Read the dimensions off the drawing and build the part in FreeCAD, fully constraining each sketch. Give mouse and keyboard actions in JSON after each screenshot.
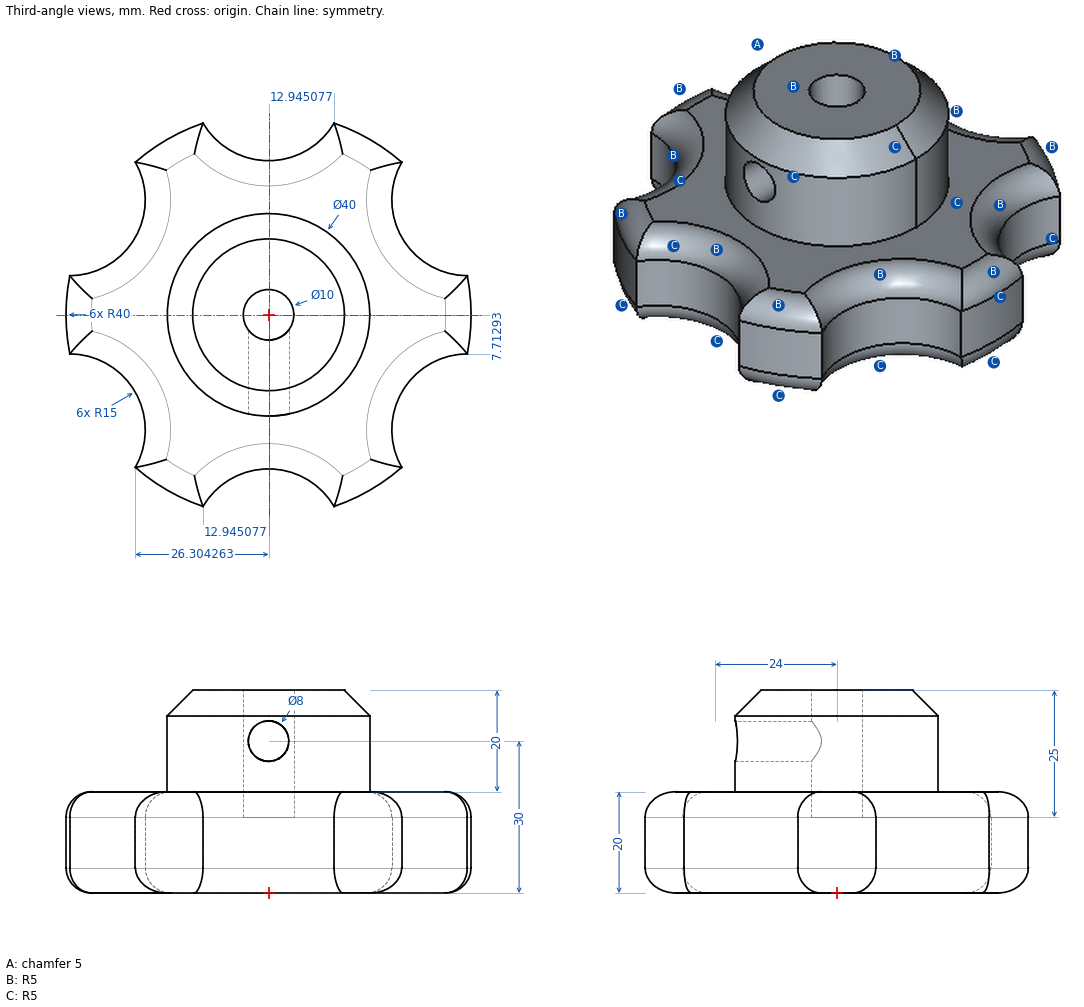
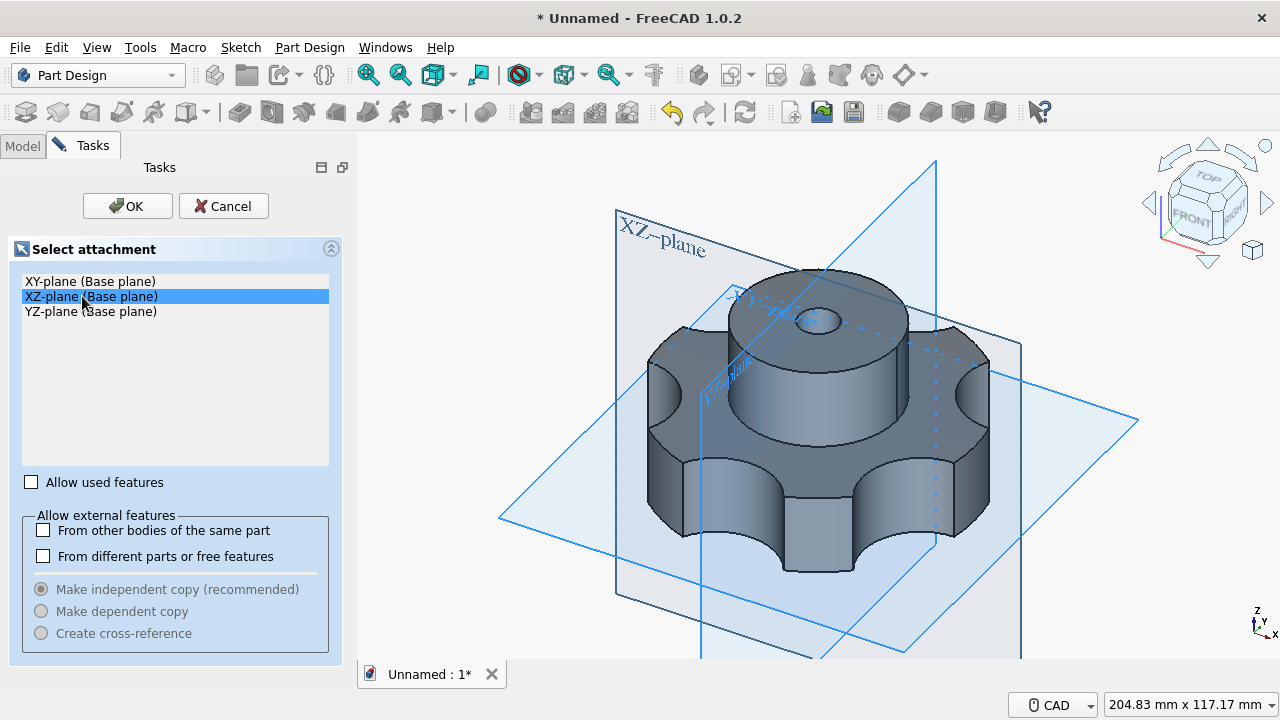
{"action": "left_click", "coordinate": [128, 206]}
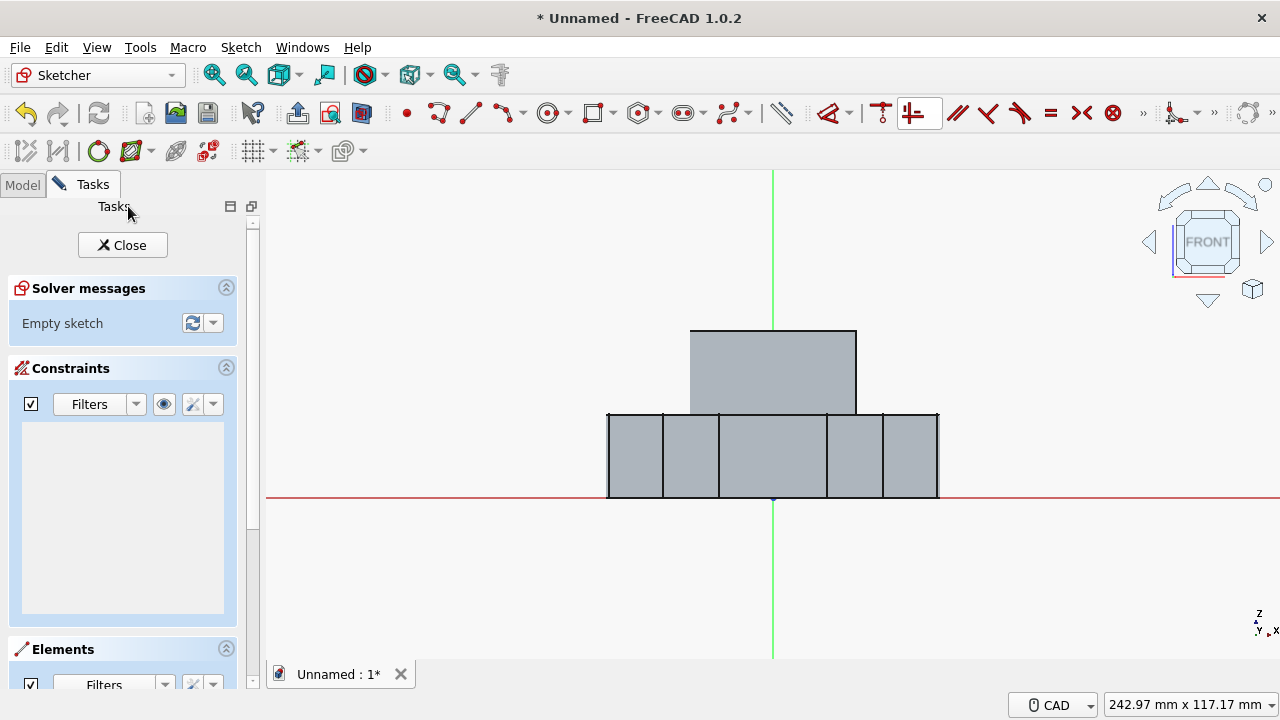
{"action": "left_click", "coordinate": [362, 114]}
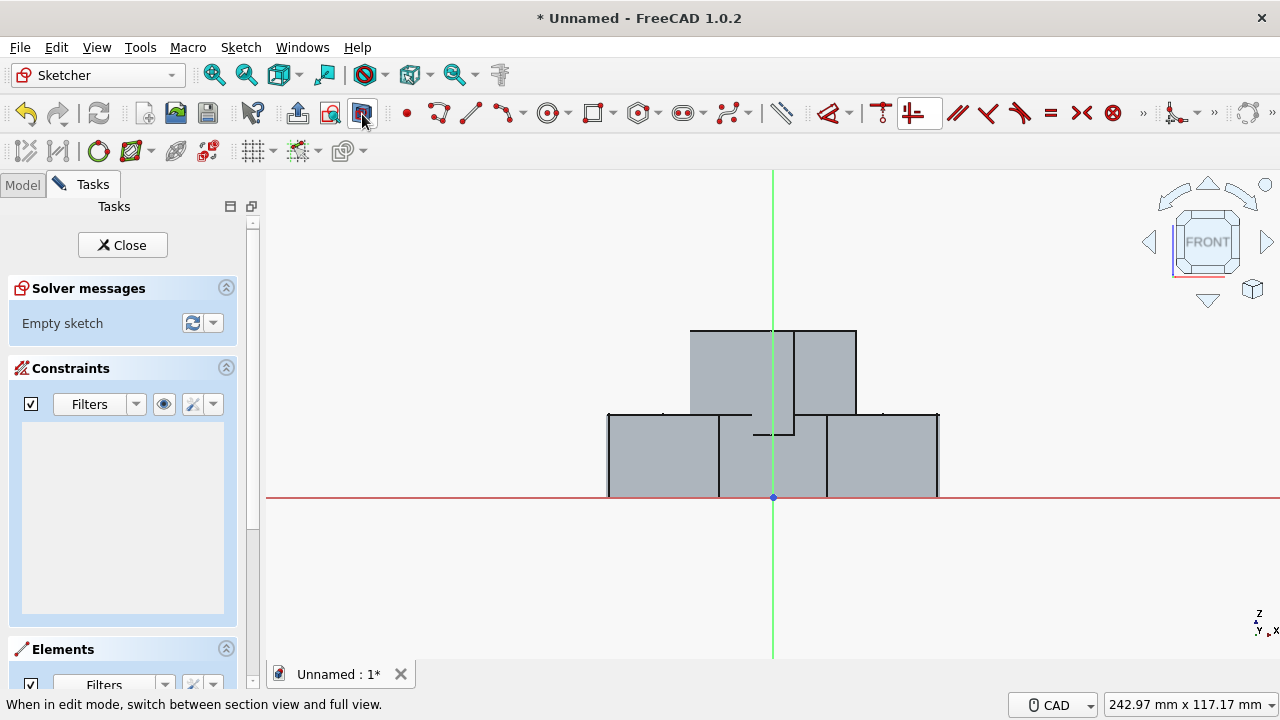
{"action": "scroll", "coordinate": [782, 368], "scroll_direction": "up", "scroll_amount": 11}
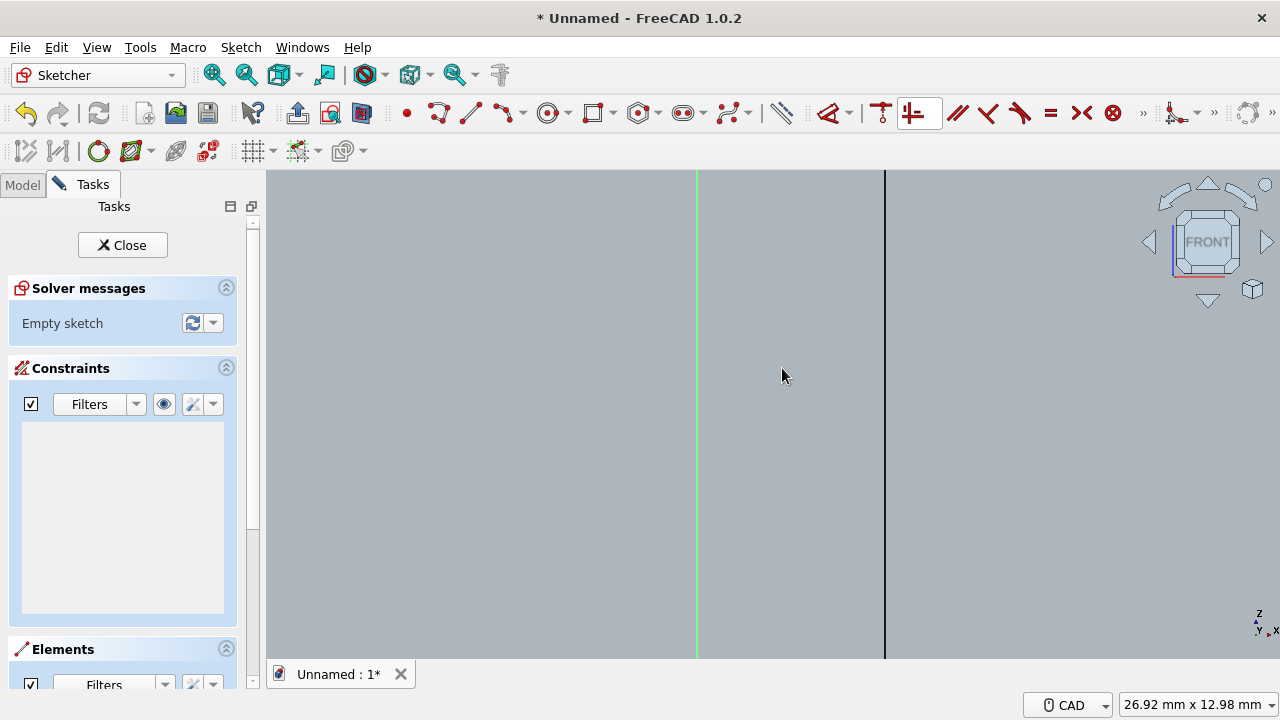
{"action": "left_click", "coordinate": [548, 114]}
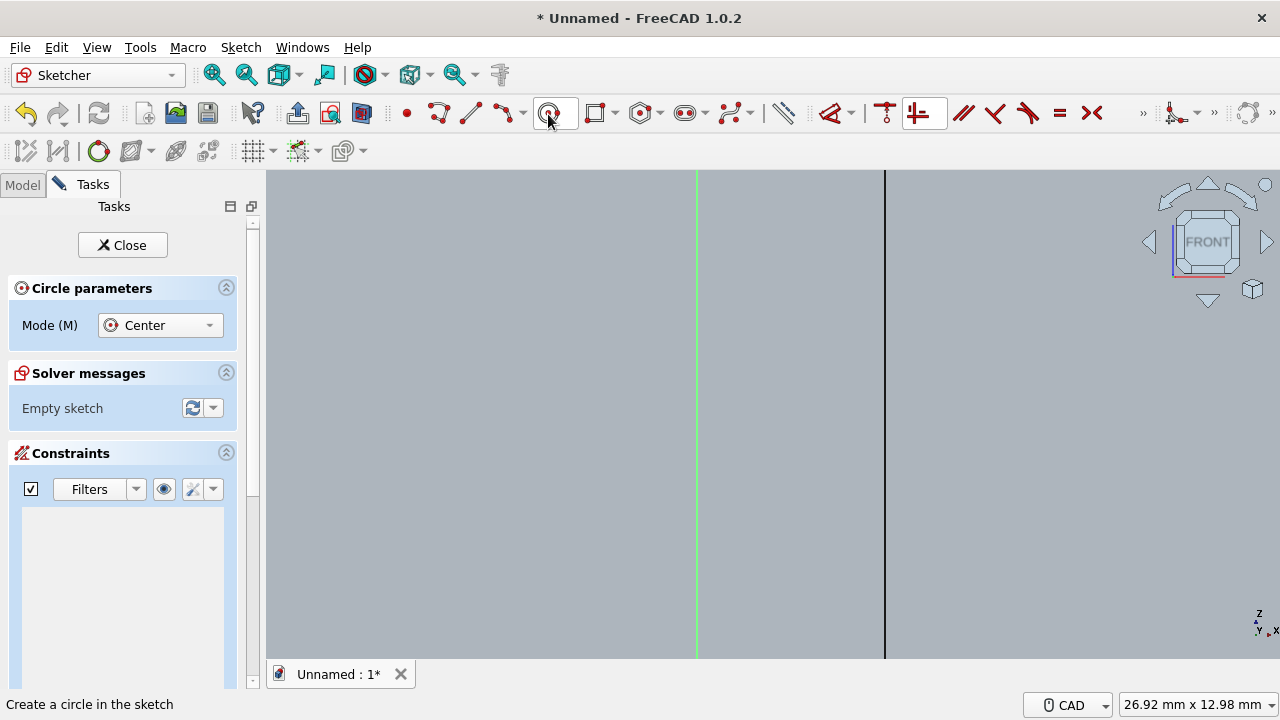
{"action": "left_click", "coordinate": [697, 408]}
{"action": "mouse_move", "coordinate": [803, 301]}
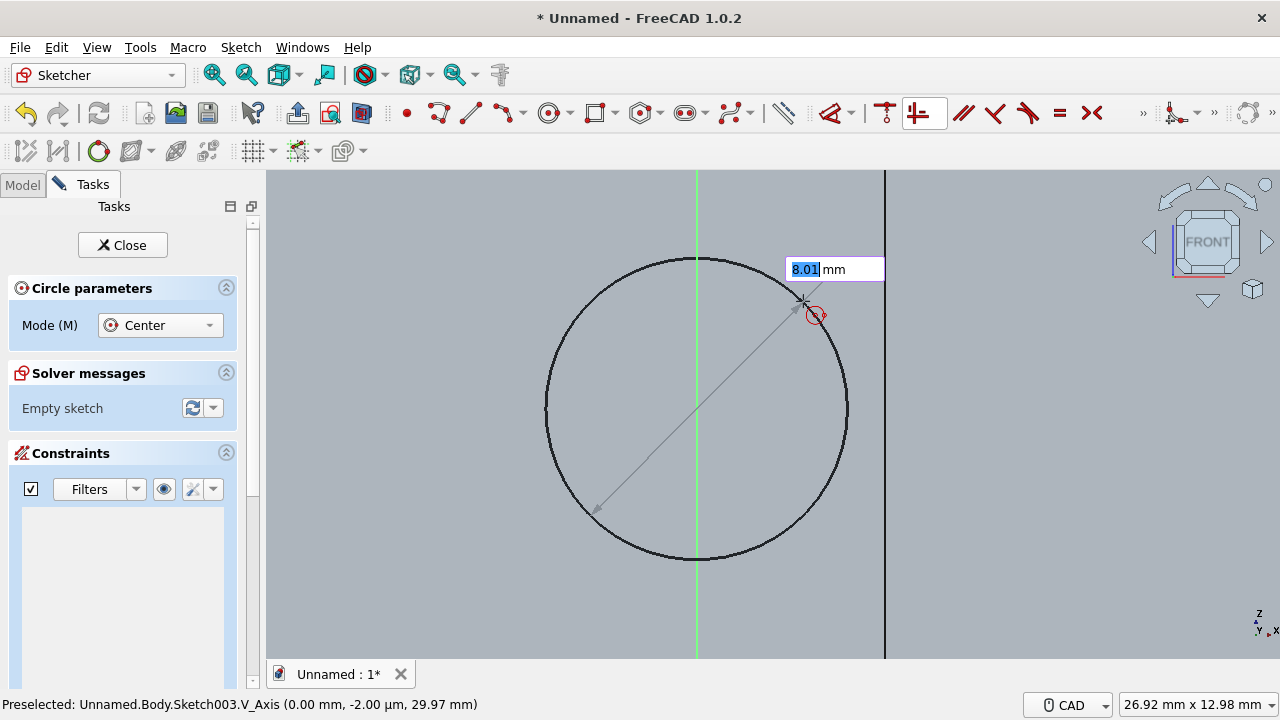
{"action": "type", "text": "8"}
{"action": "key", "text": "Return"}
{"action": "key", "text": "Escape"}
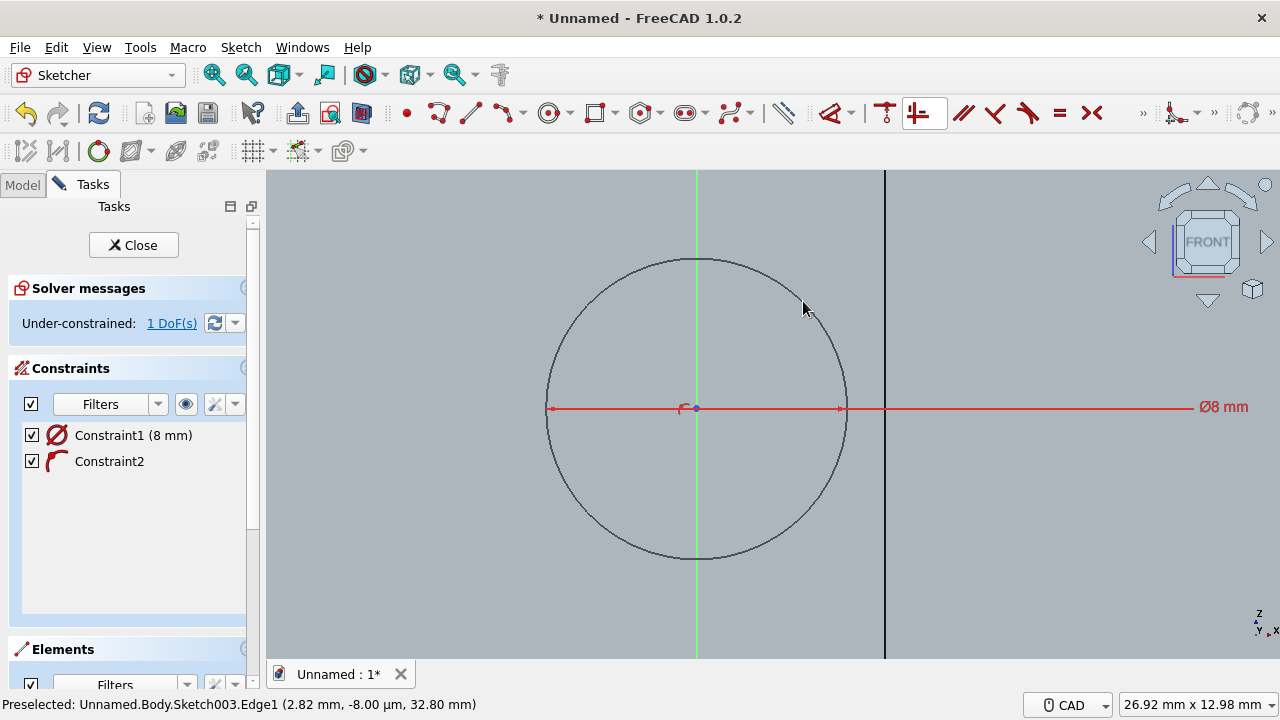
{"action": "left_click", "coordinate": [830, 114]}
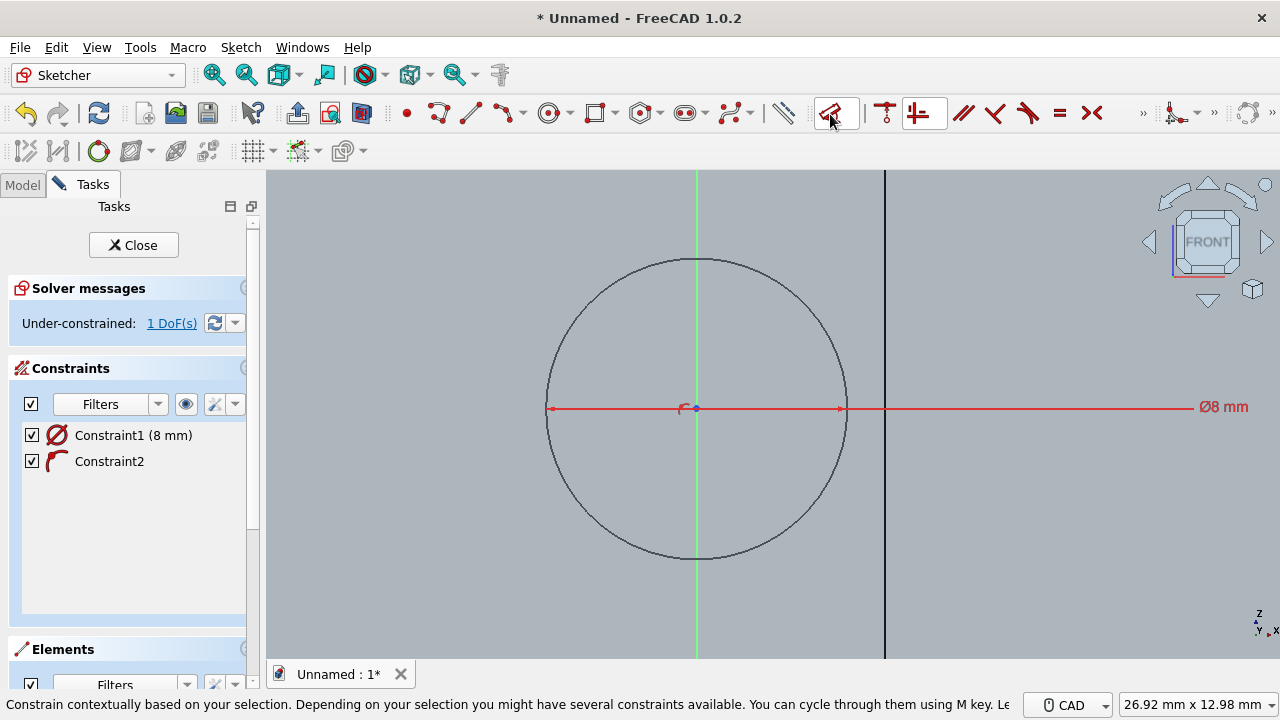
{"action": "left_click", "coordinate": [697, 409]}
{"action": "left_click", "coordinate": [731, 520]}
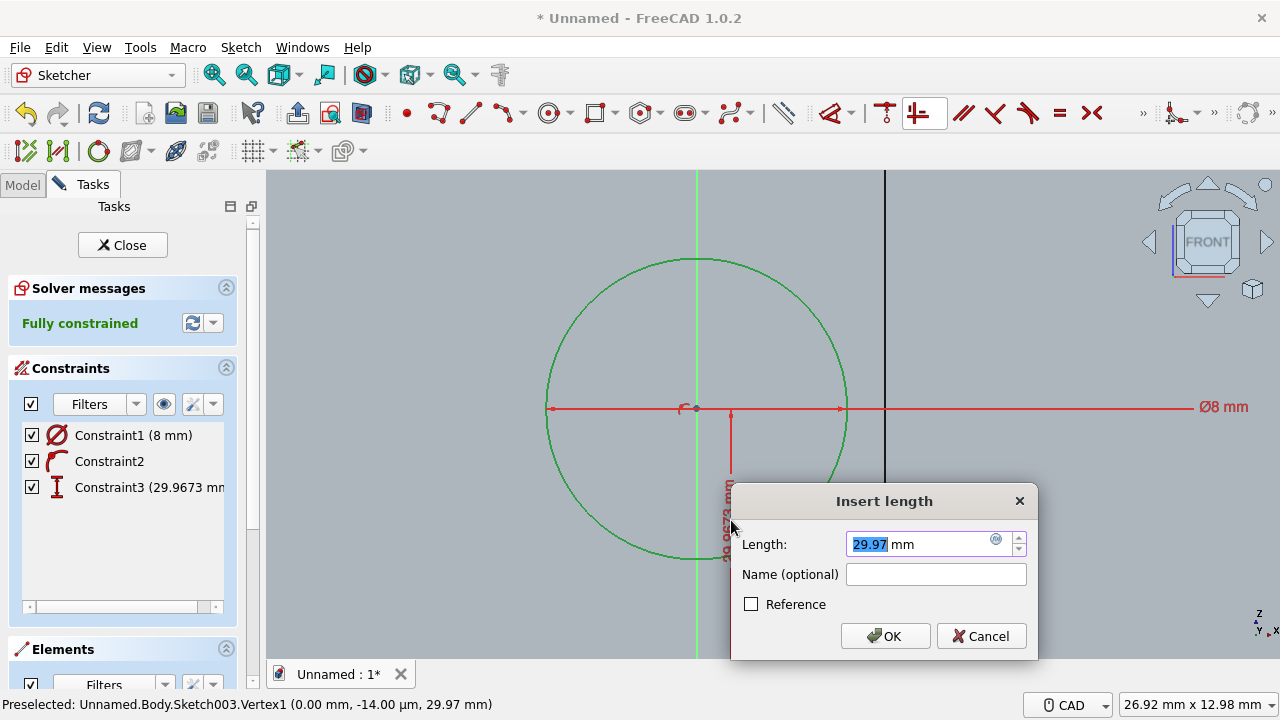
{"action": "type", "text": "30"}
{"action": "key", "text": "Return"}
{"action": "key", "text": "Escape"}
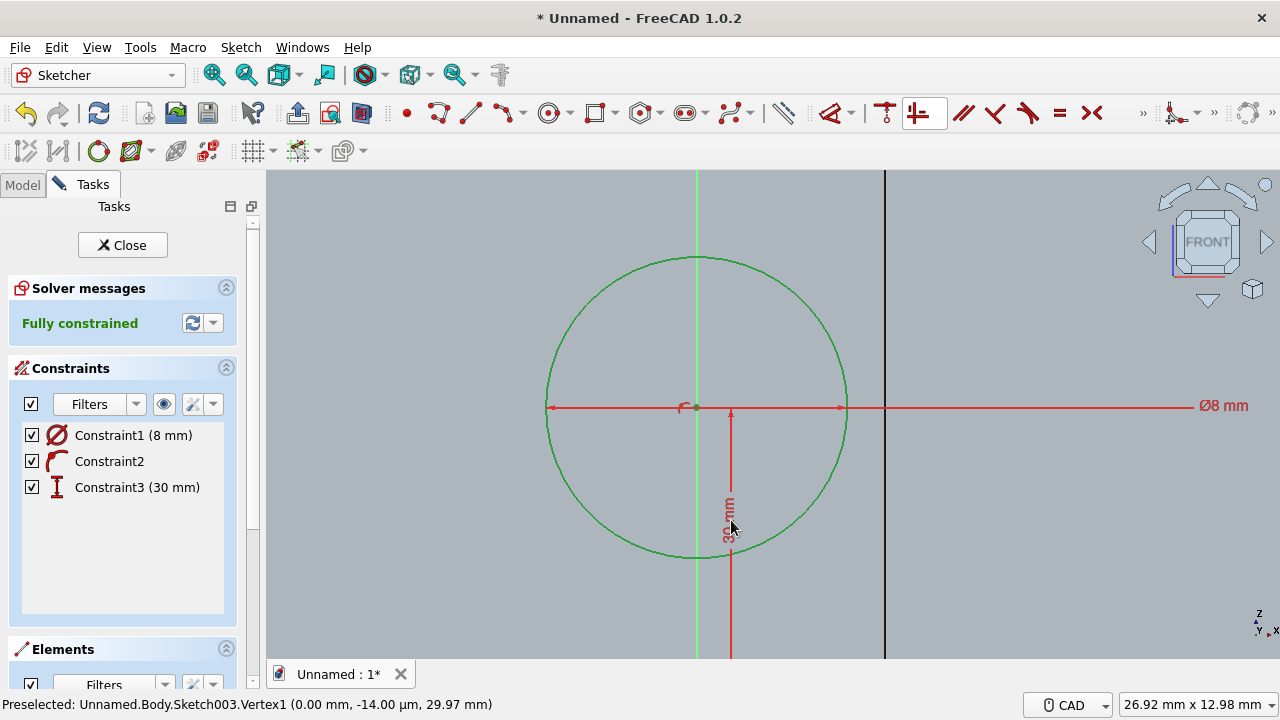
{"action": "left_click", "coordinate": [123, 245]}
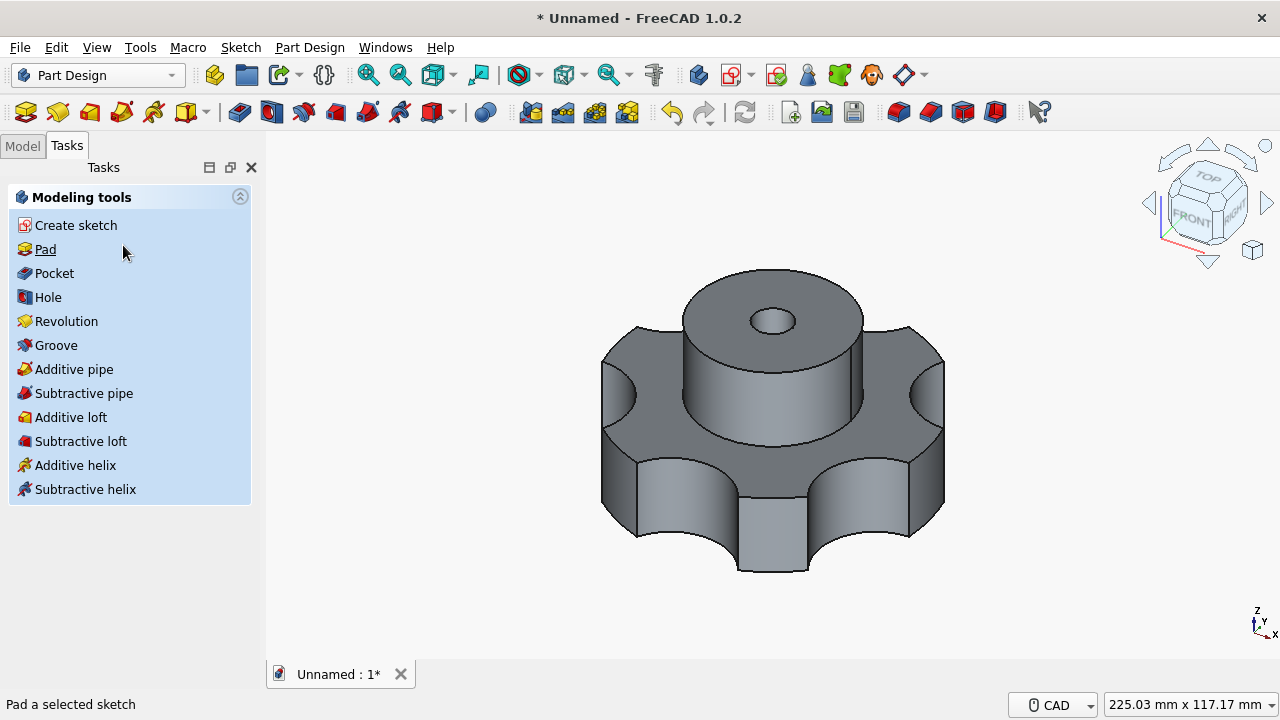
{"action": "left_click", "coordinate": [240, 112]}